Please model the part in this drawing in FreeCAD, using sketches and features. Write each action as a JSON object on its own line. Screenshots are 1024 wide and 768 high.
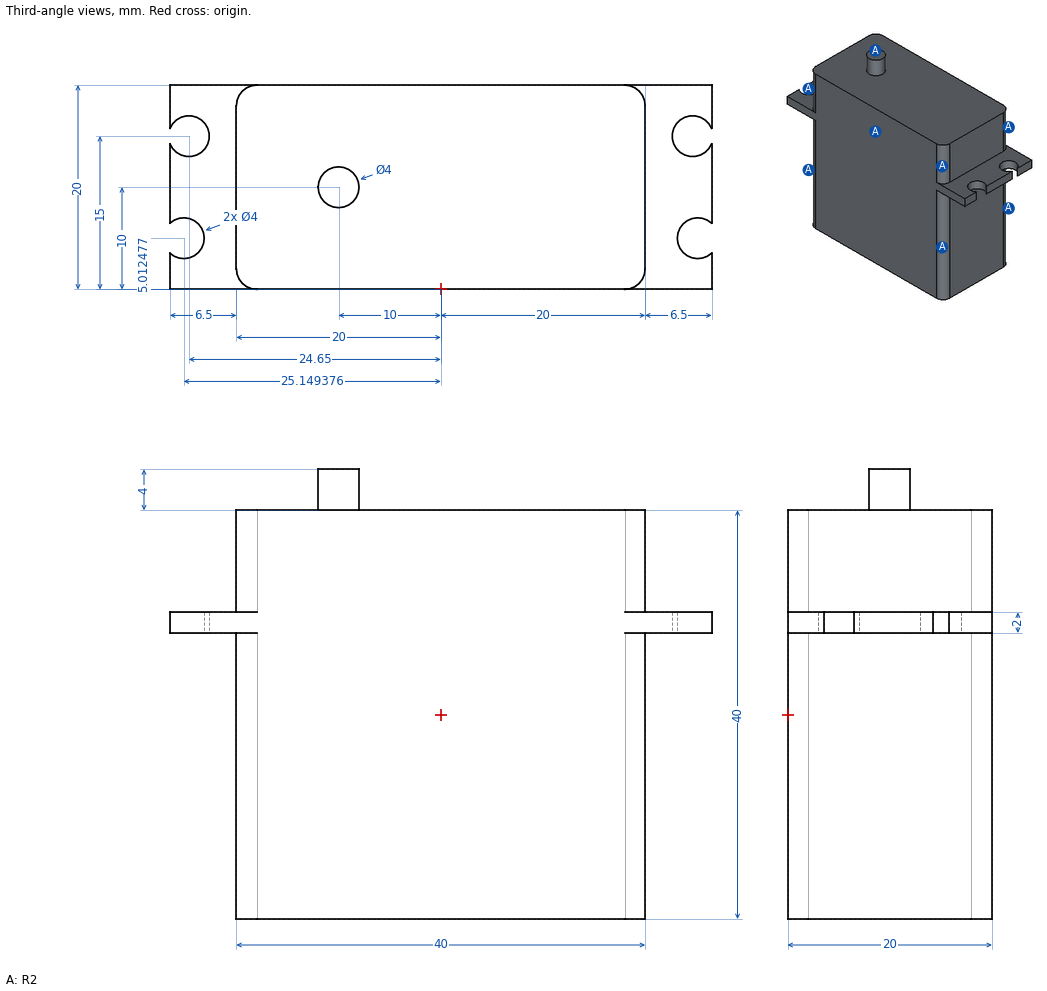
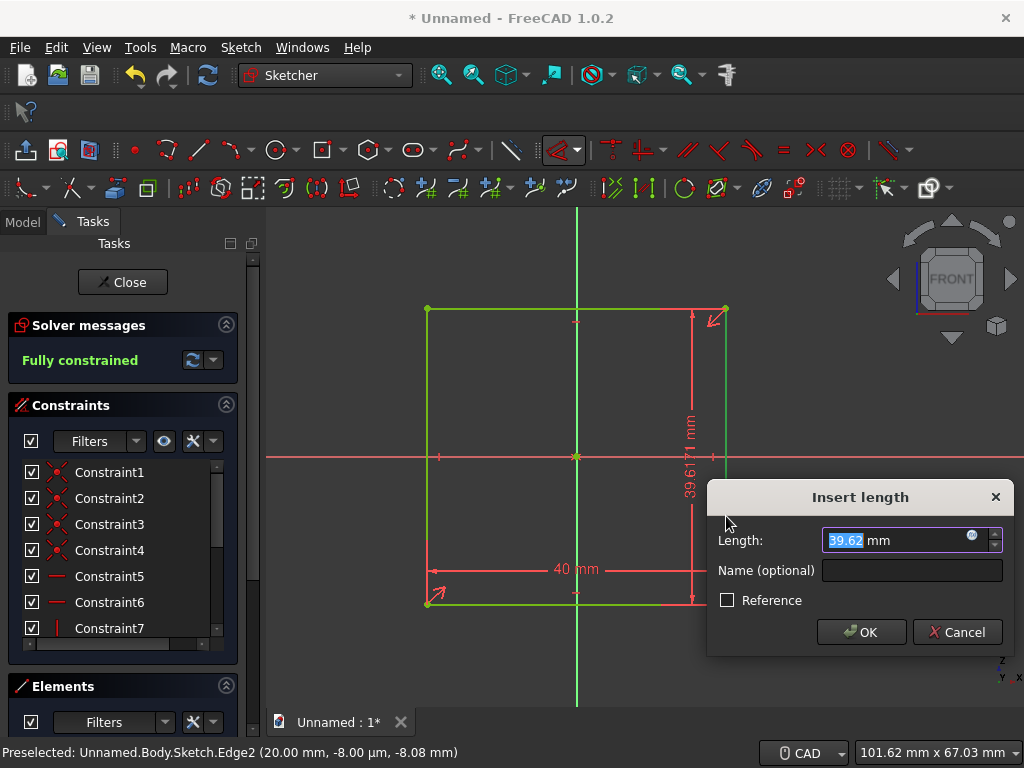
{"action": "type", "text": "40"}
{"action": "key", "text": "Return"}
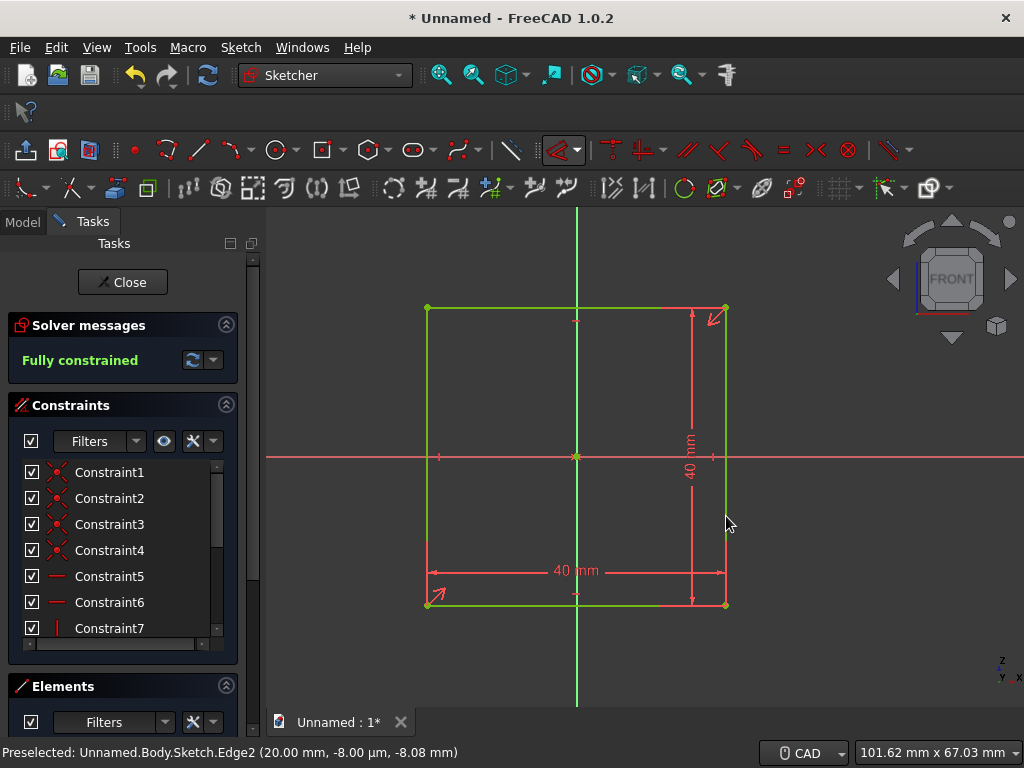
{"action": "left_click", "coordinate": [123, 282]}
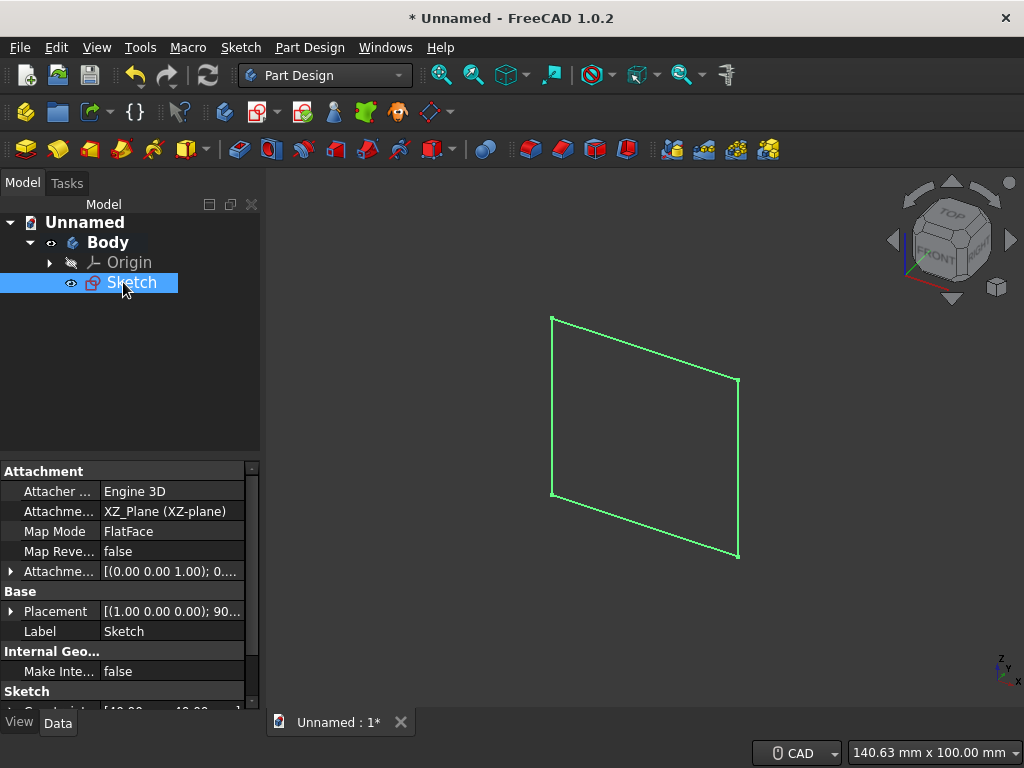
{"action": "left_click", "coordinate": [26, 150]}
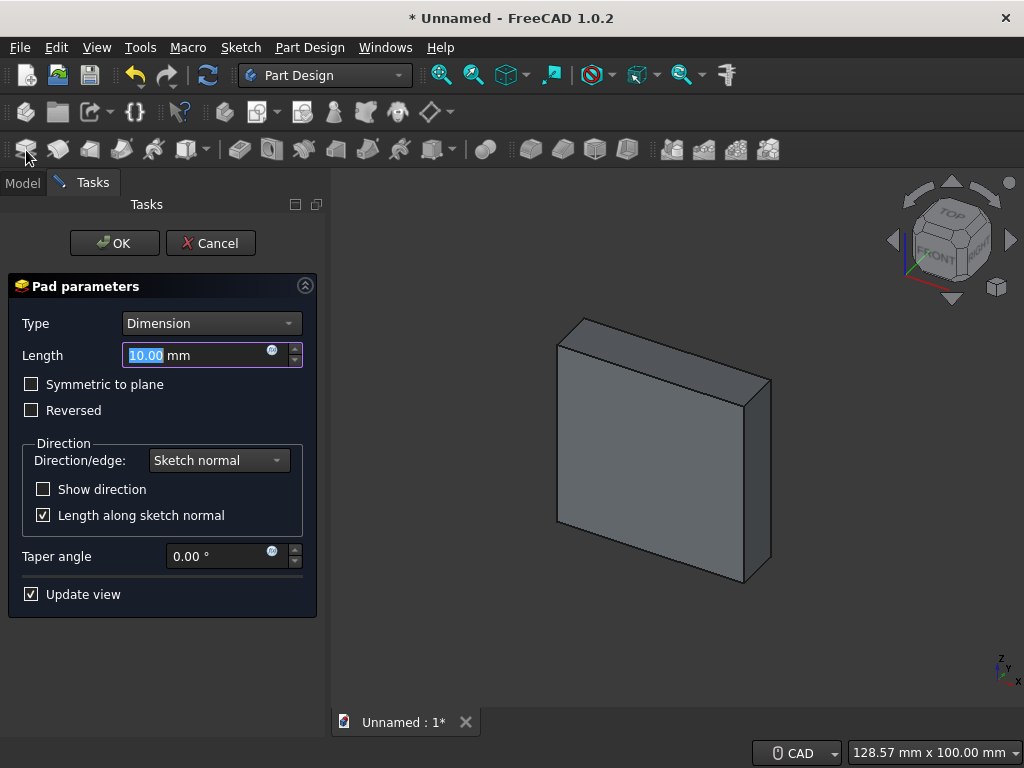
{"action": "type", "text": "20"}
{"action": "key", "text": "Tab"}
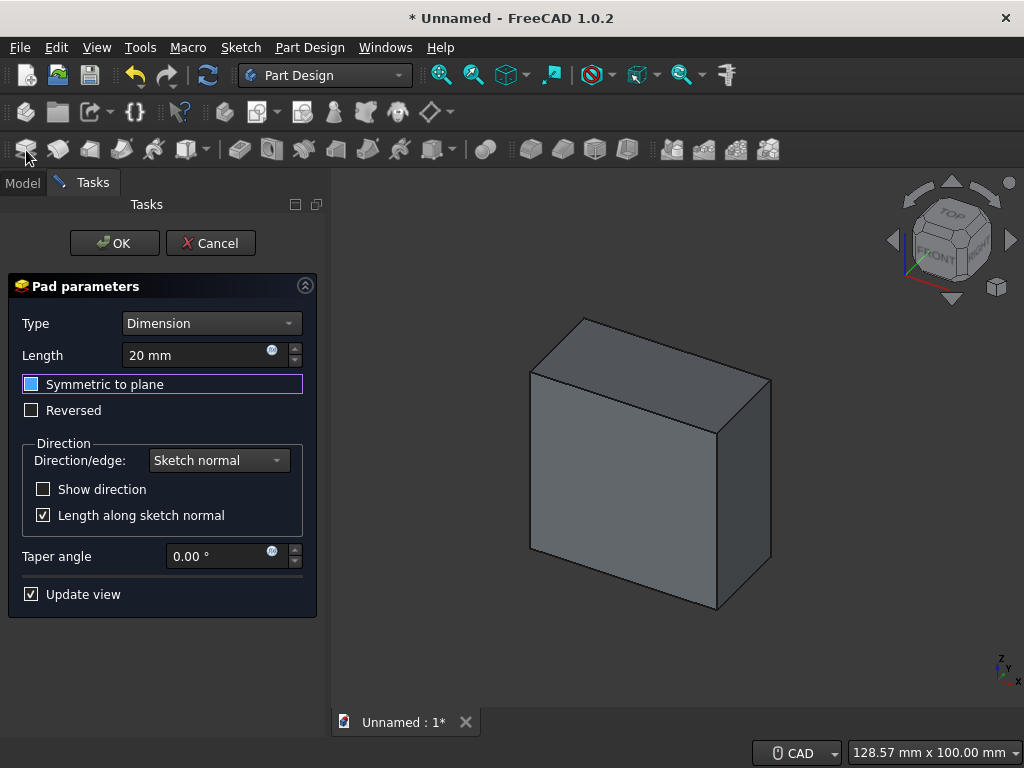
{"action": "left_click", "coordinate": [30, 410]}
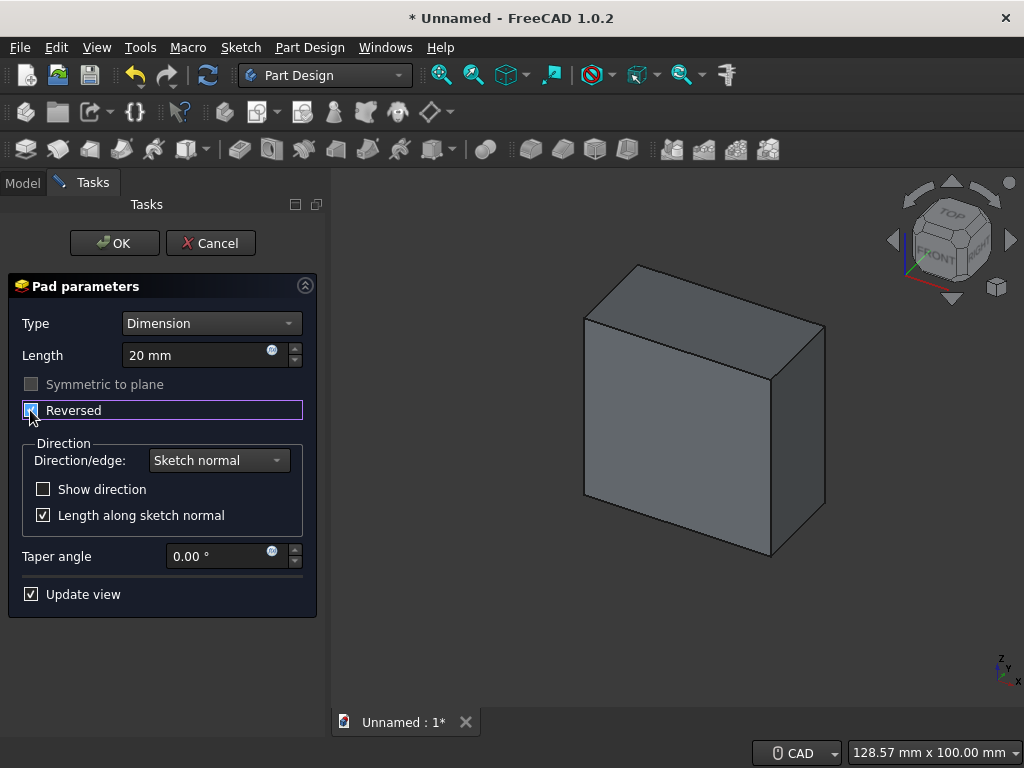
{"action": "left_click", "coordinate": [115, 243]}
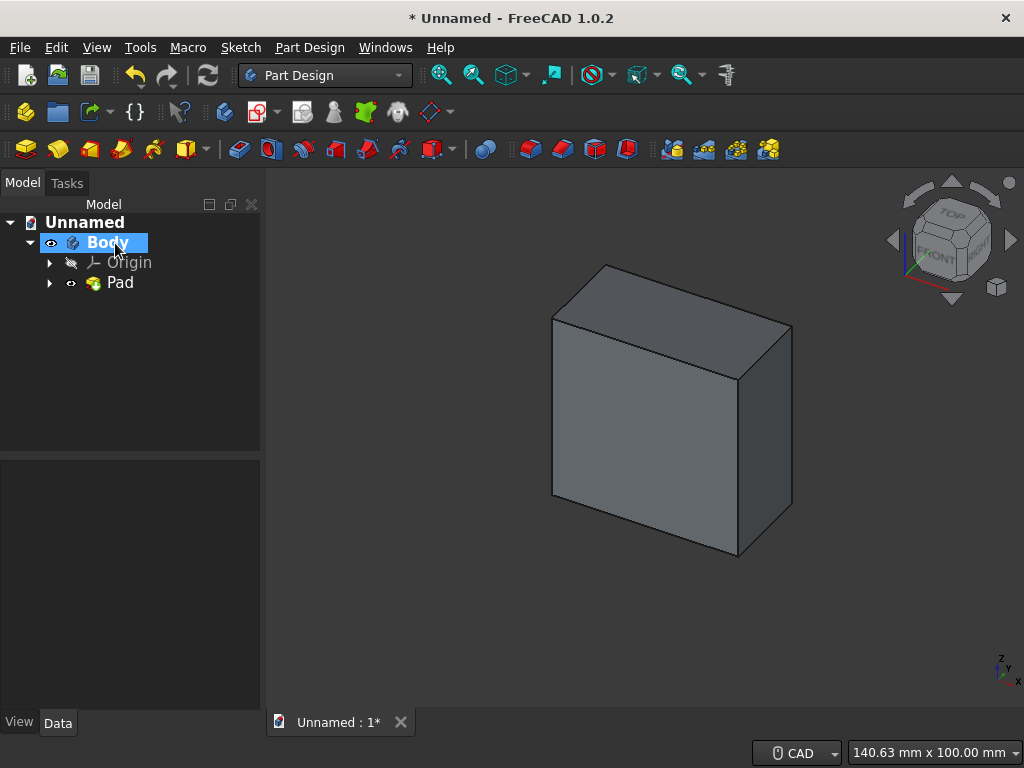
{"action": "left_click", "coordinate": [50, 263]}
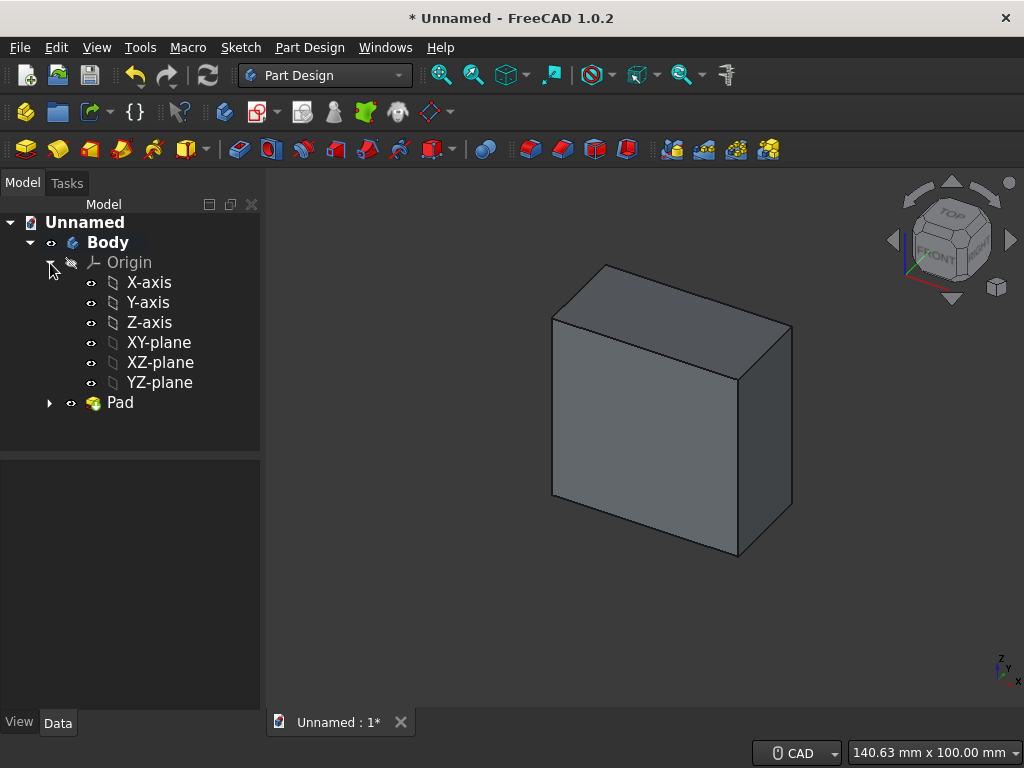
{"action": "left_click", "coordinate": [136, 343]}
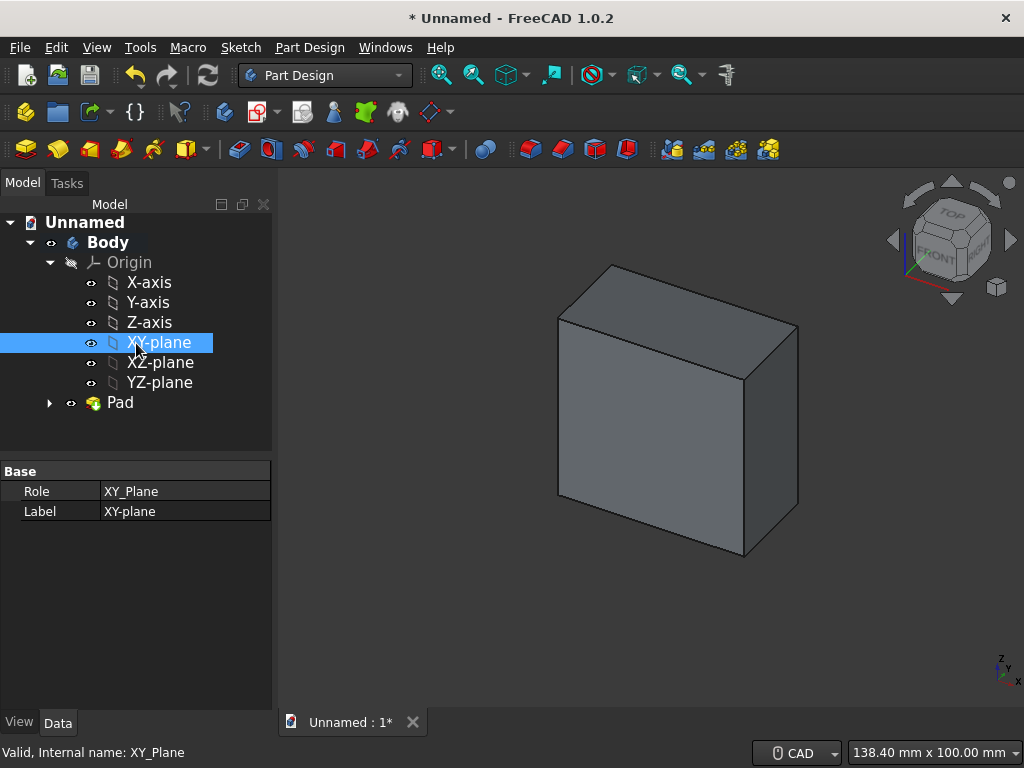
{"action": "left_click", "coordinate": [430, 112]}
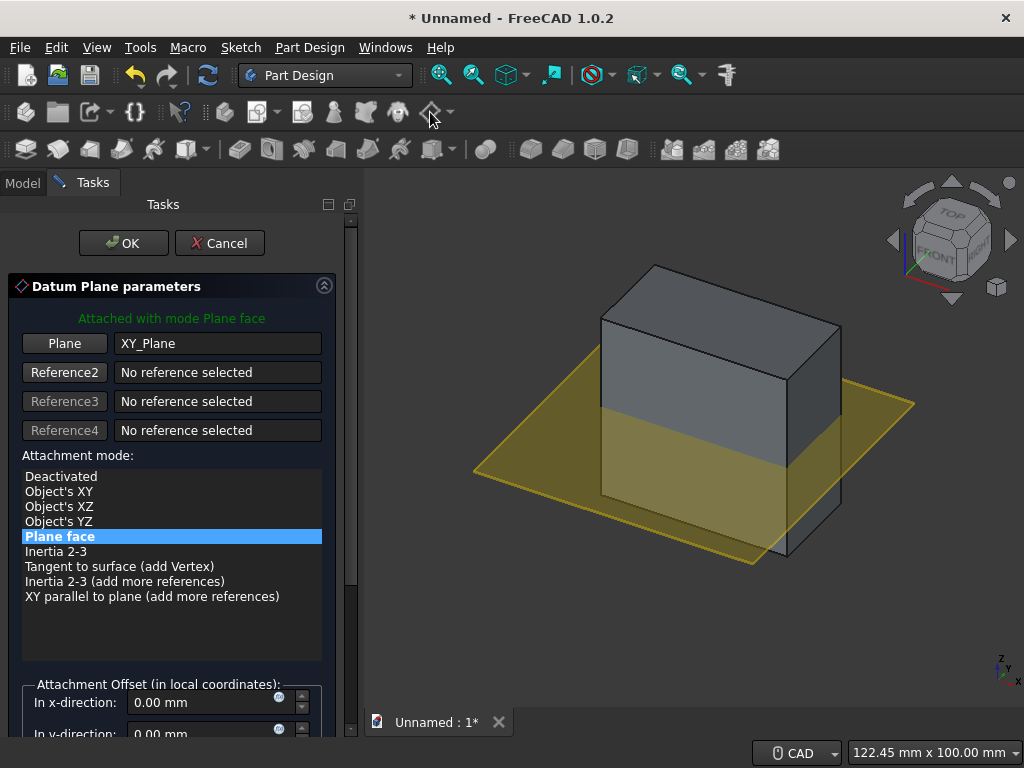
{"action": "scroll", "coordinate": [351, 475], "scroll_direction": "down", "scroll_amount": 2}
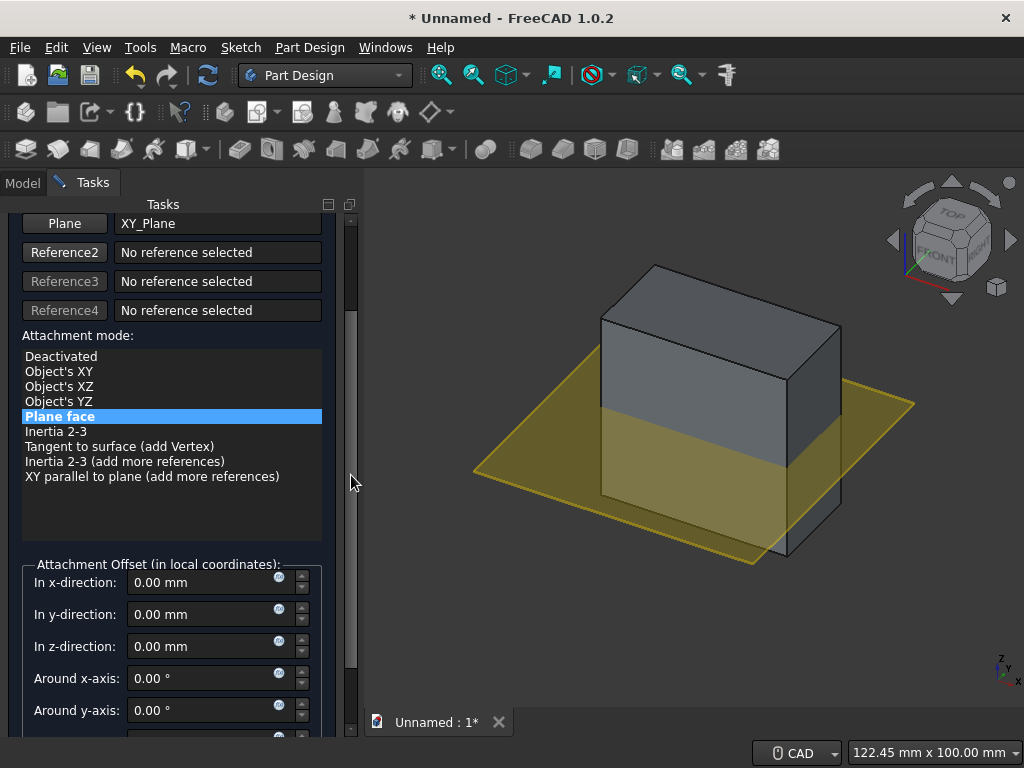
{"action": "triple_click", "coordinate": [210, 646]}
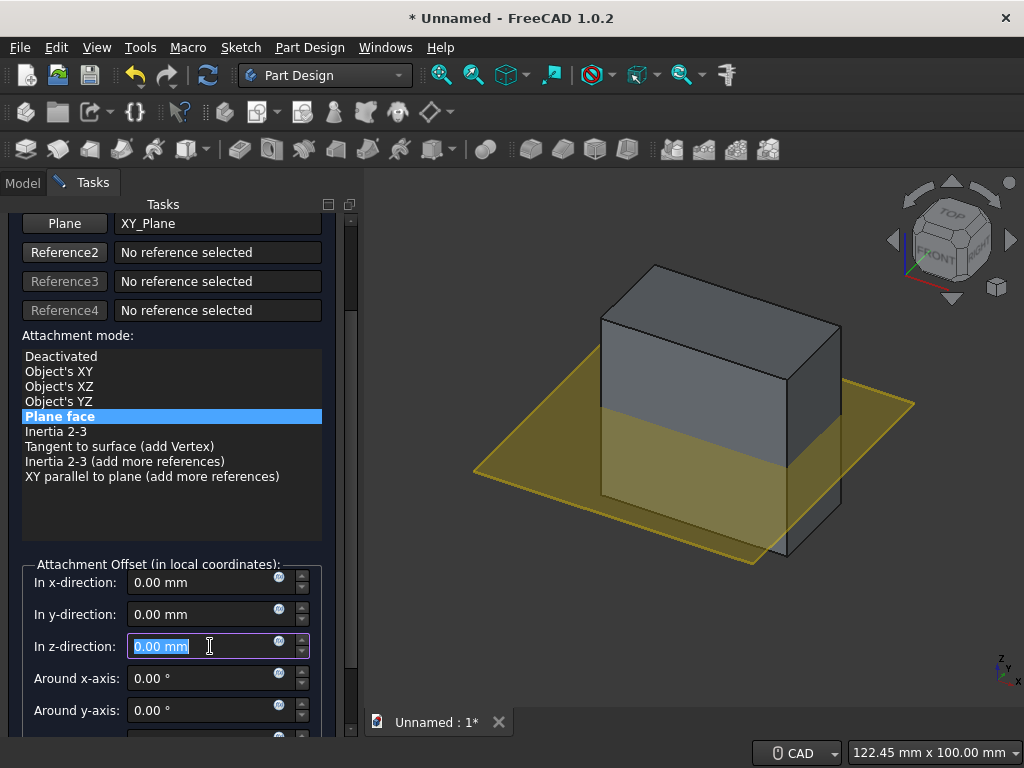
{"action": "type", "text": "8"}
{"action": "key", "text": "Tab"}